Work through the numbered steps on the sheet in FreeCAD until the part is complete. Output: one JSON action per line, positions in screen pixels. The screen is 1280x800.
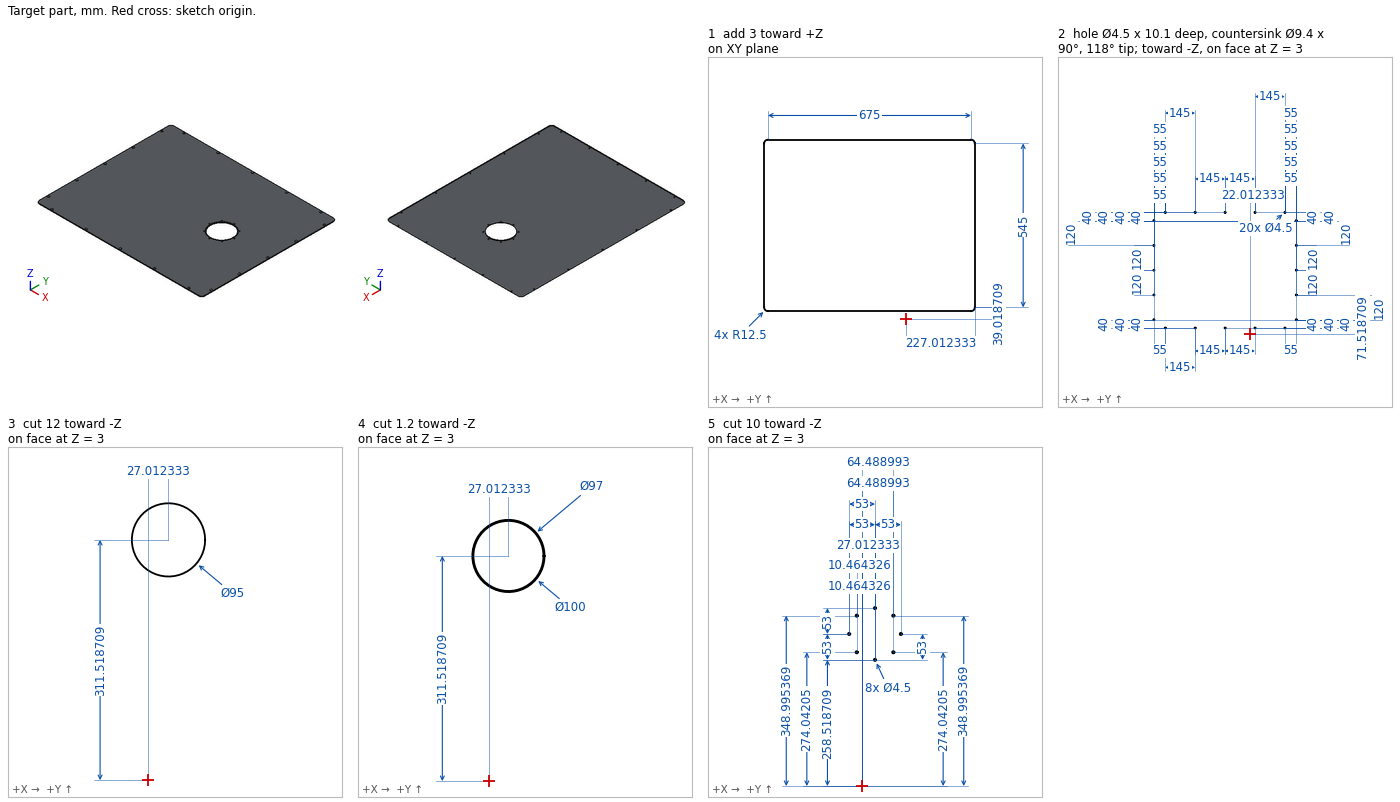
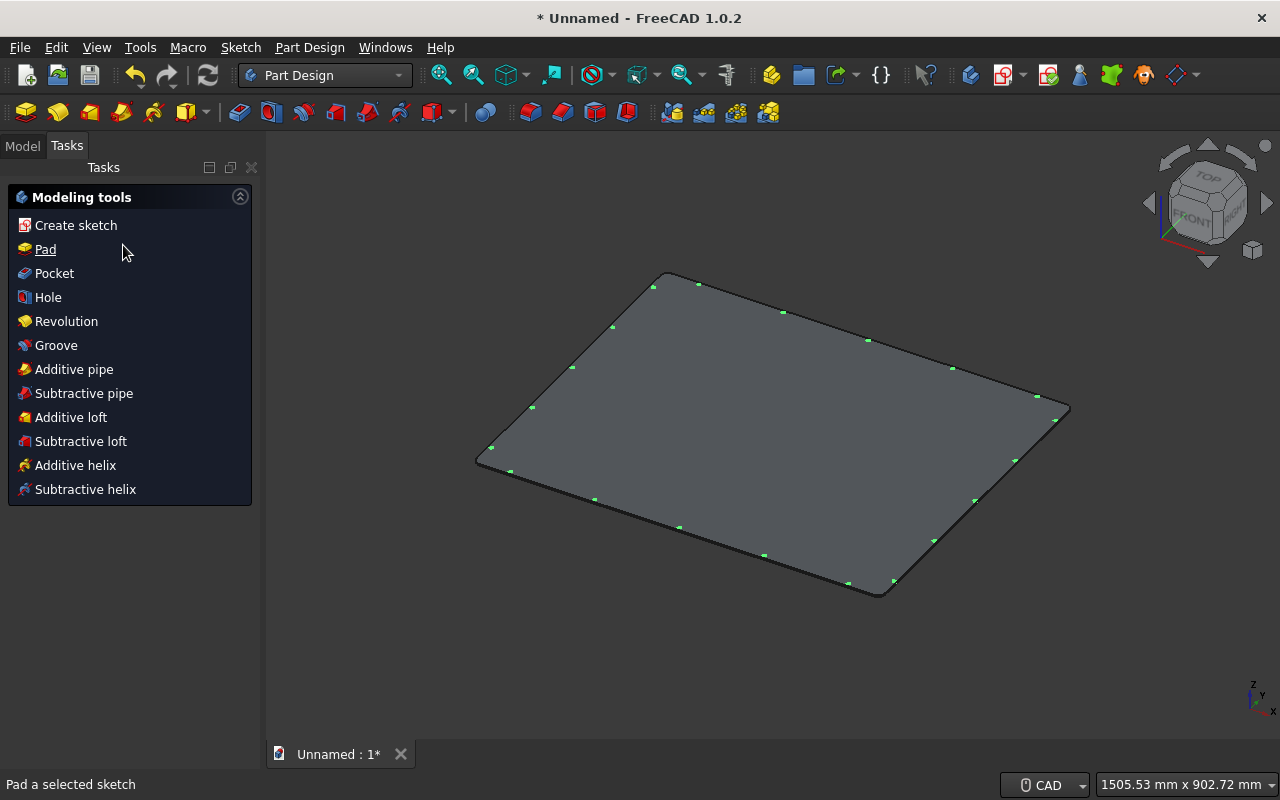
{"action": "left_click", "coordinate": [272, 112]}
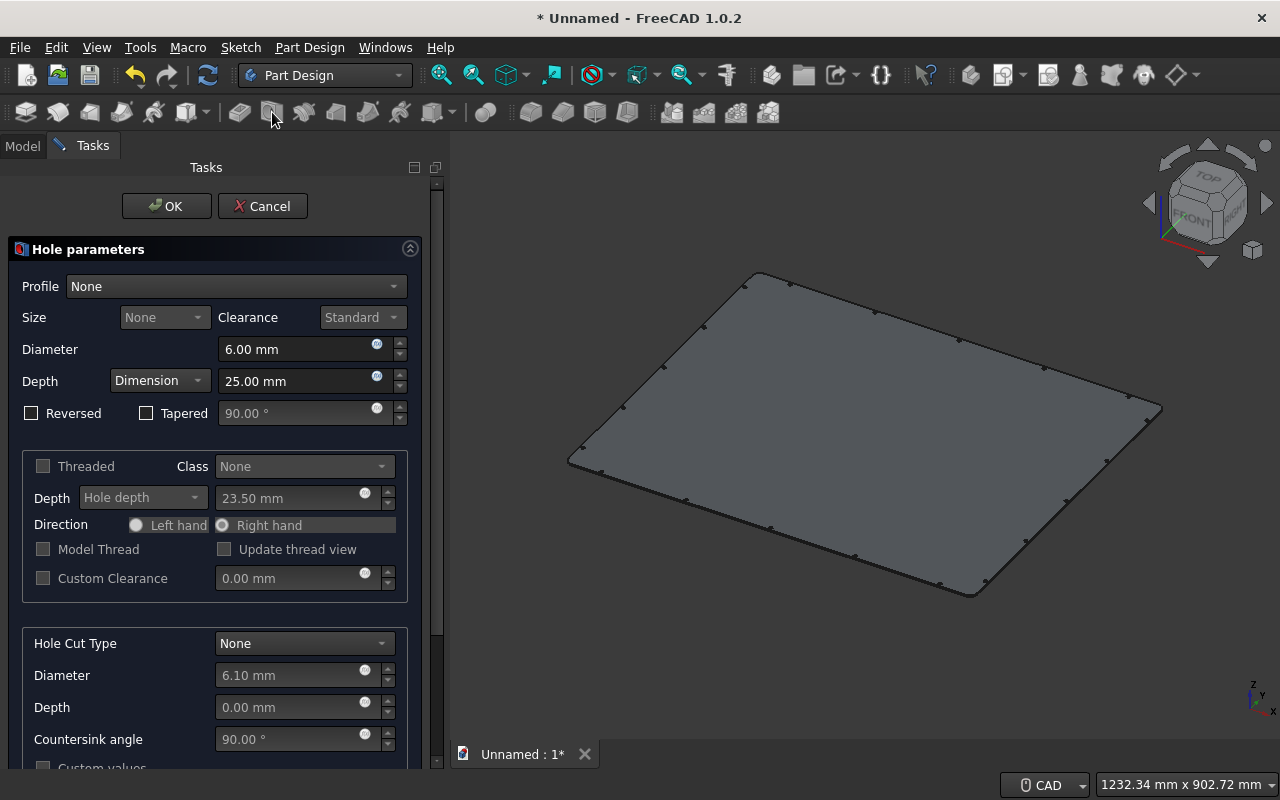
{"action": "triple_click", "coordinate": [305, 349]}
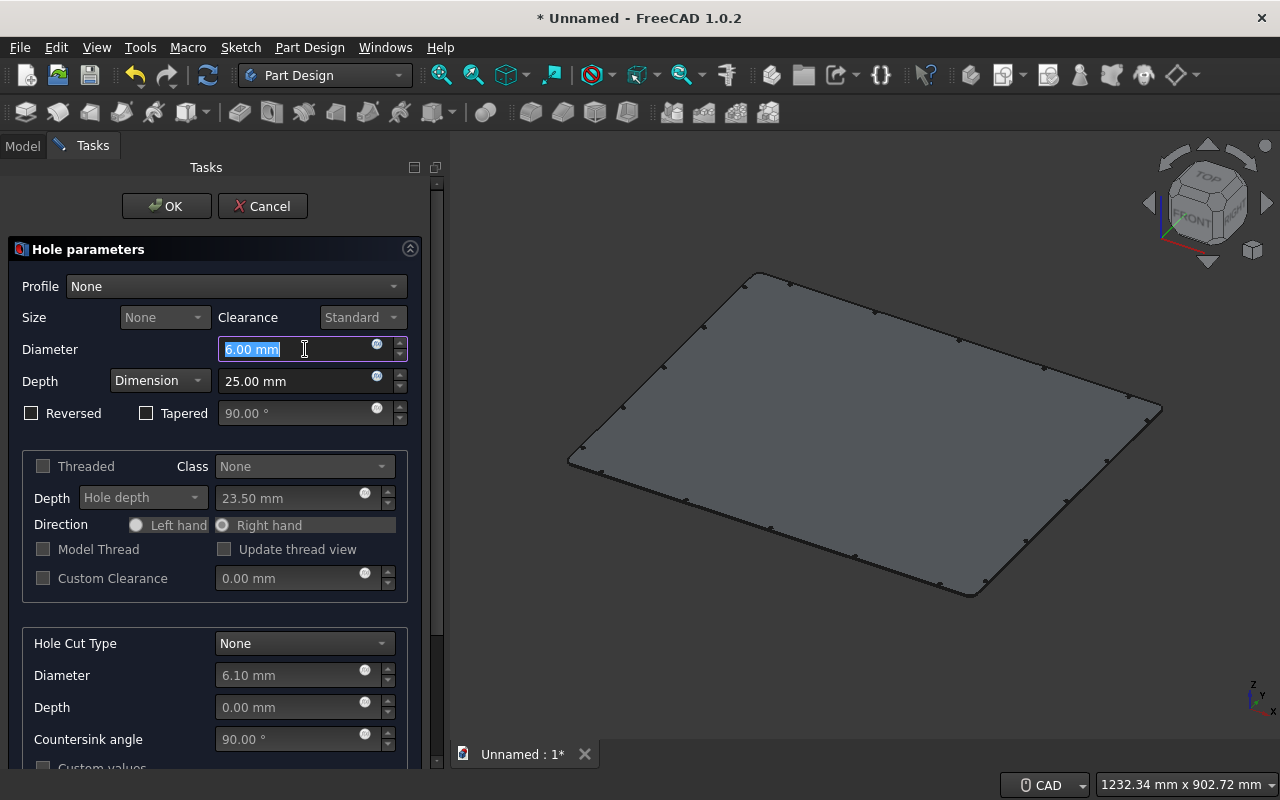
{"action": "type", "text": "4.5"}
{"action": "key", "text": "Tab"}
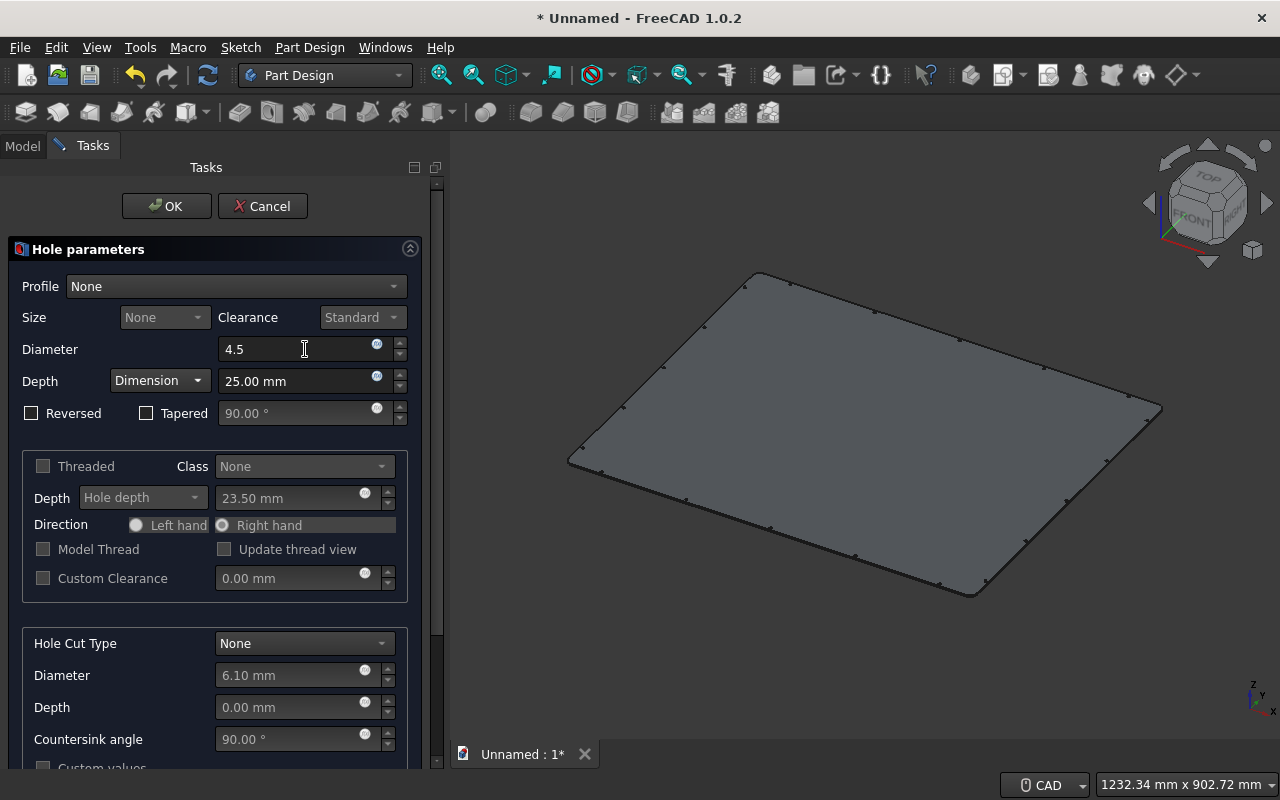
{"action": "triple_click", "coordinate": [305, 381]}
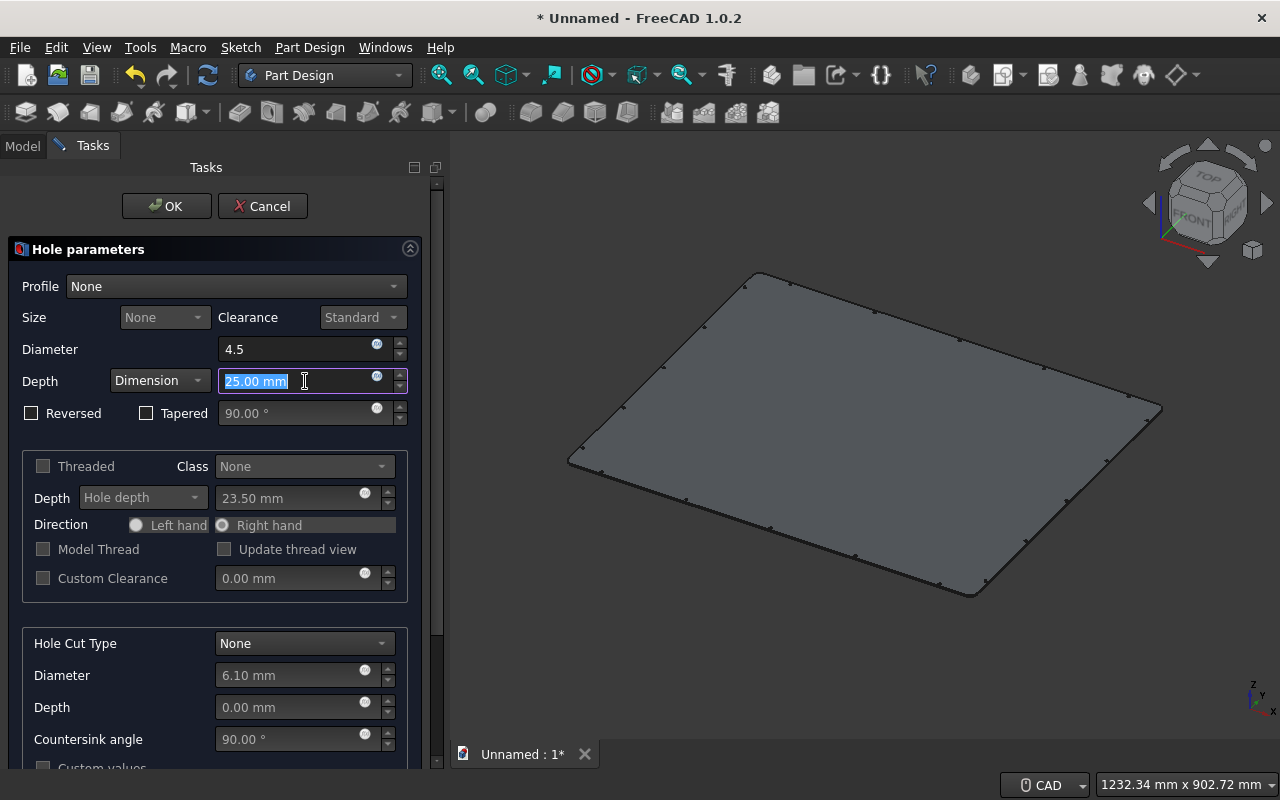
{"action": "type", "text": "10.1"}
{"action": "key", "text": "Tab"}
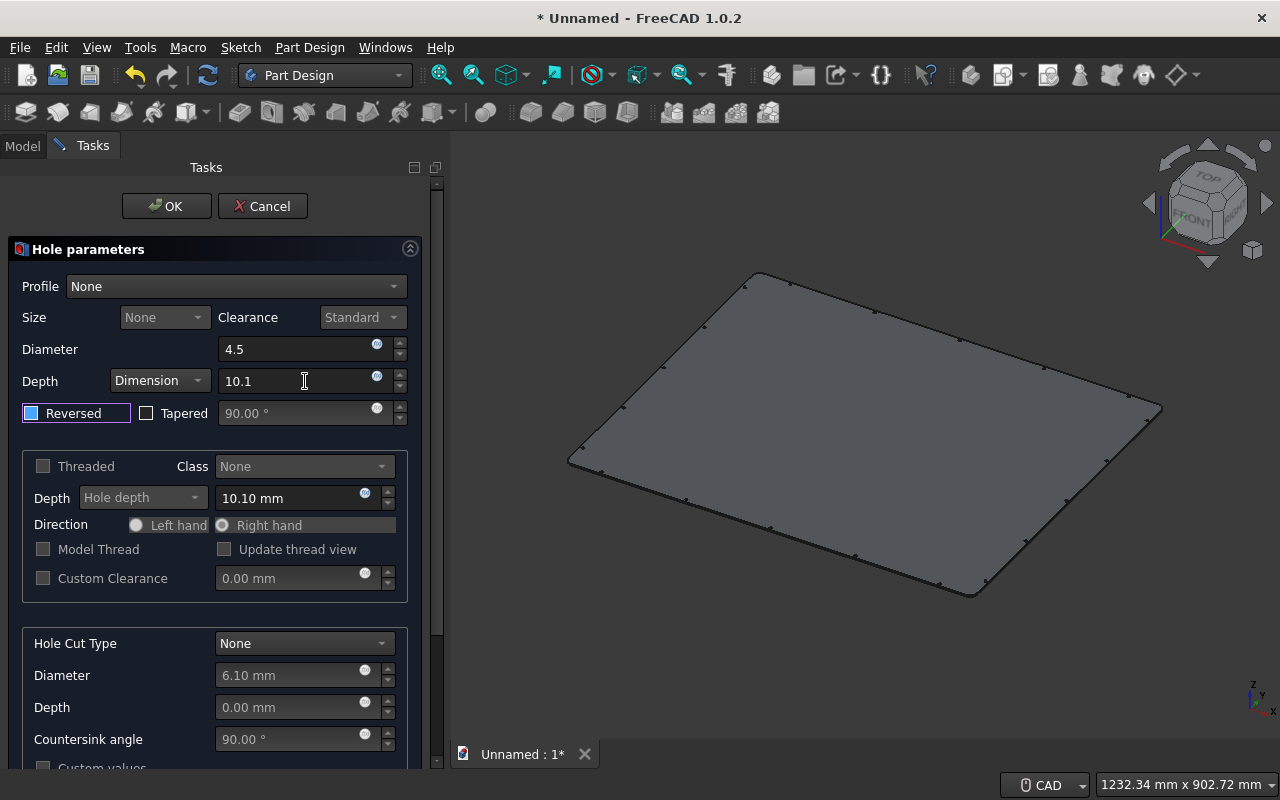
{"action": "left_click", "coordinate": [306, 644]}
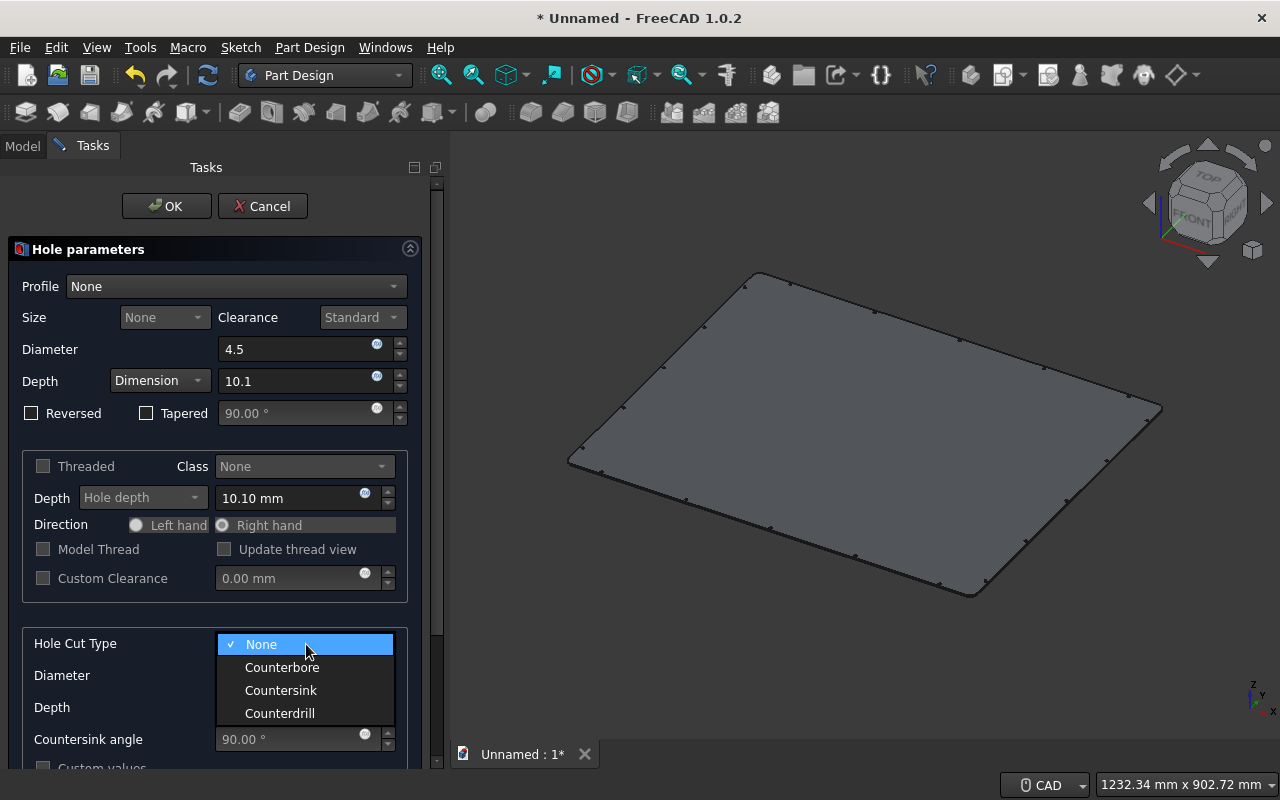
{"action": "left_click", "coordinate": [304, 690]}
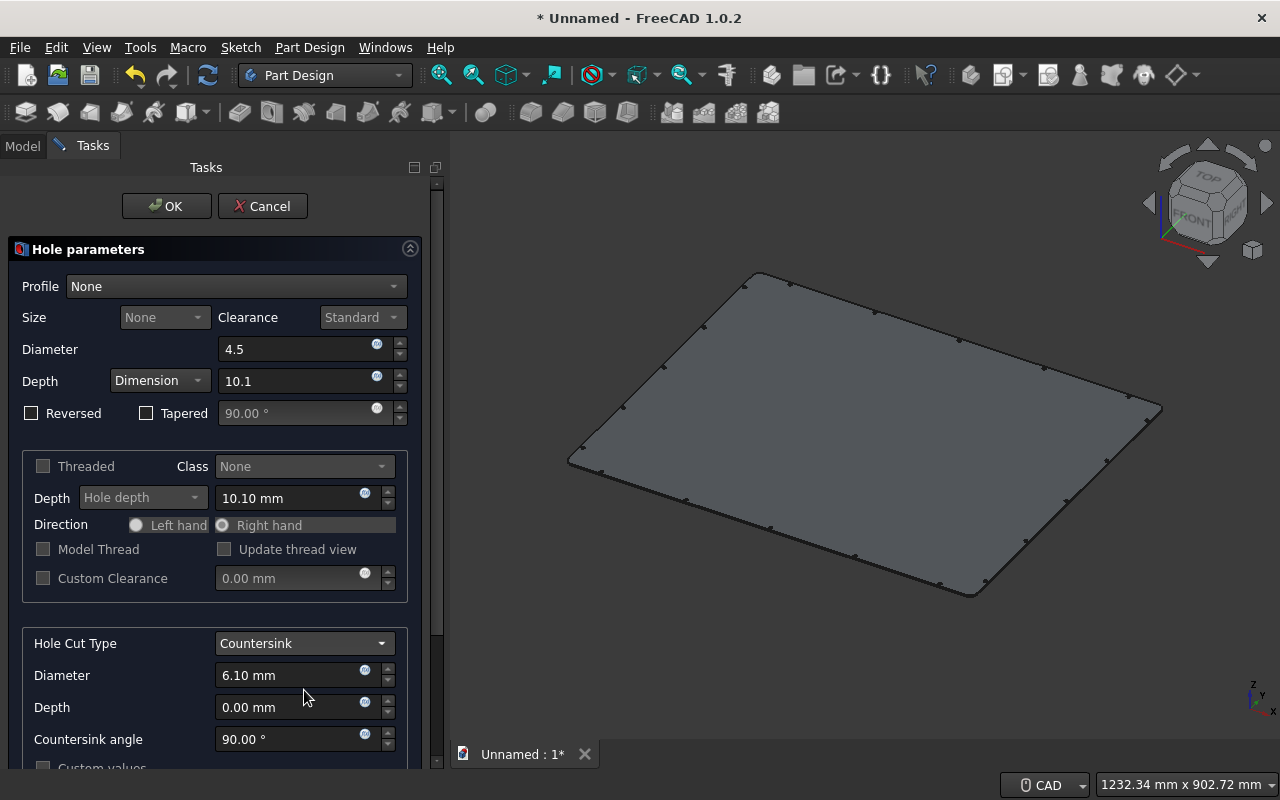
{"action": "triple_click", "coordinate": [298, 675]}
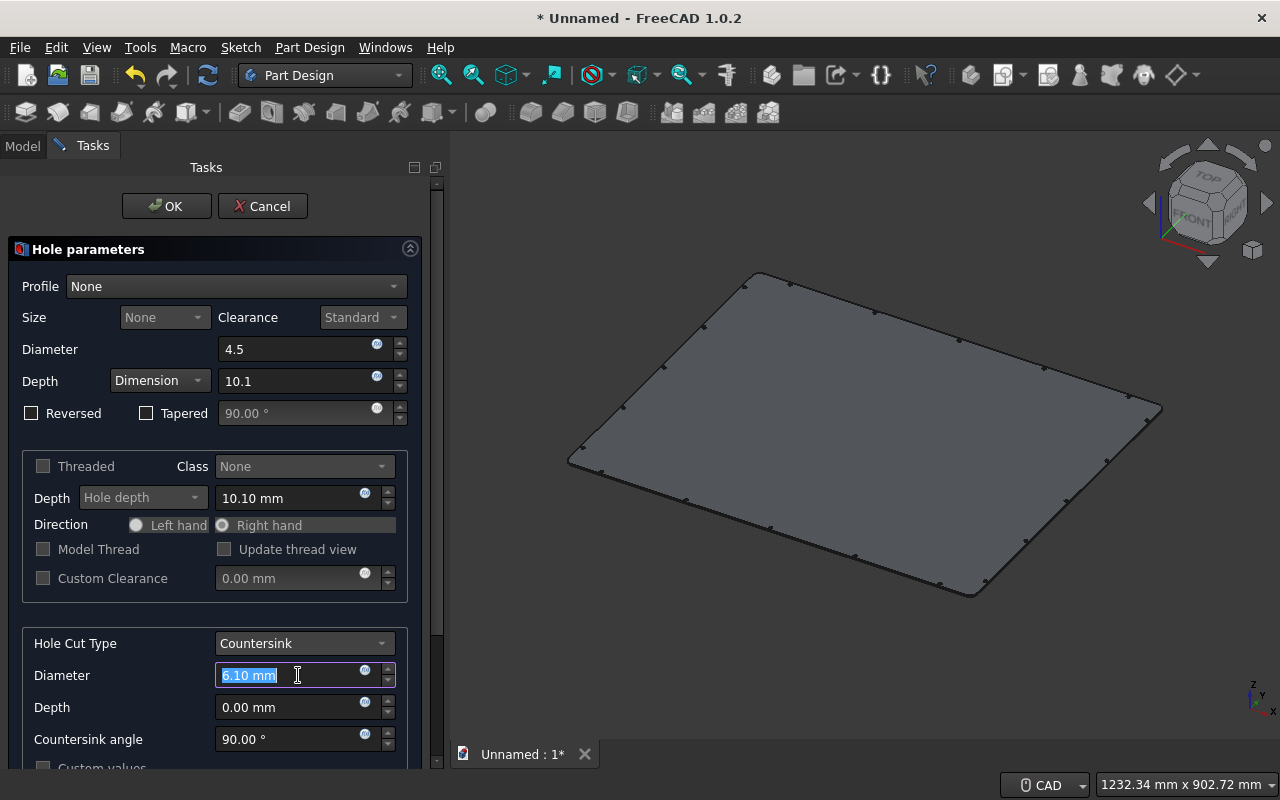
{"action": "type", "text": "9.4"}
{"action": "key", "text": "Tab"}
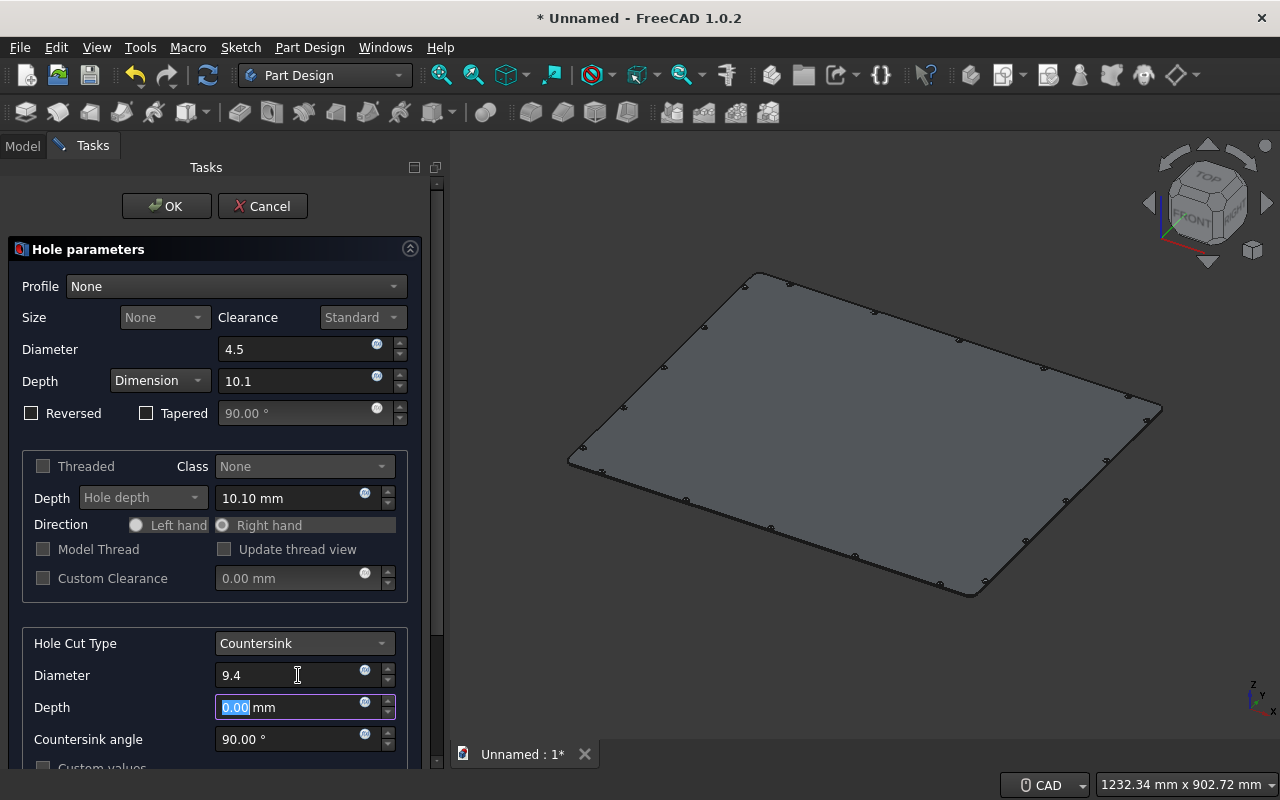
{"action": "left_click", "coordinate": [167, 206]}